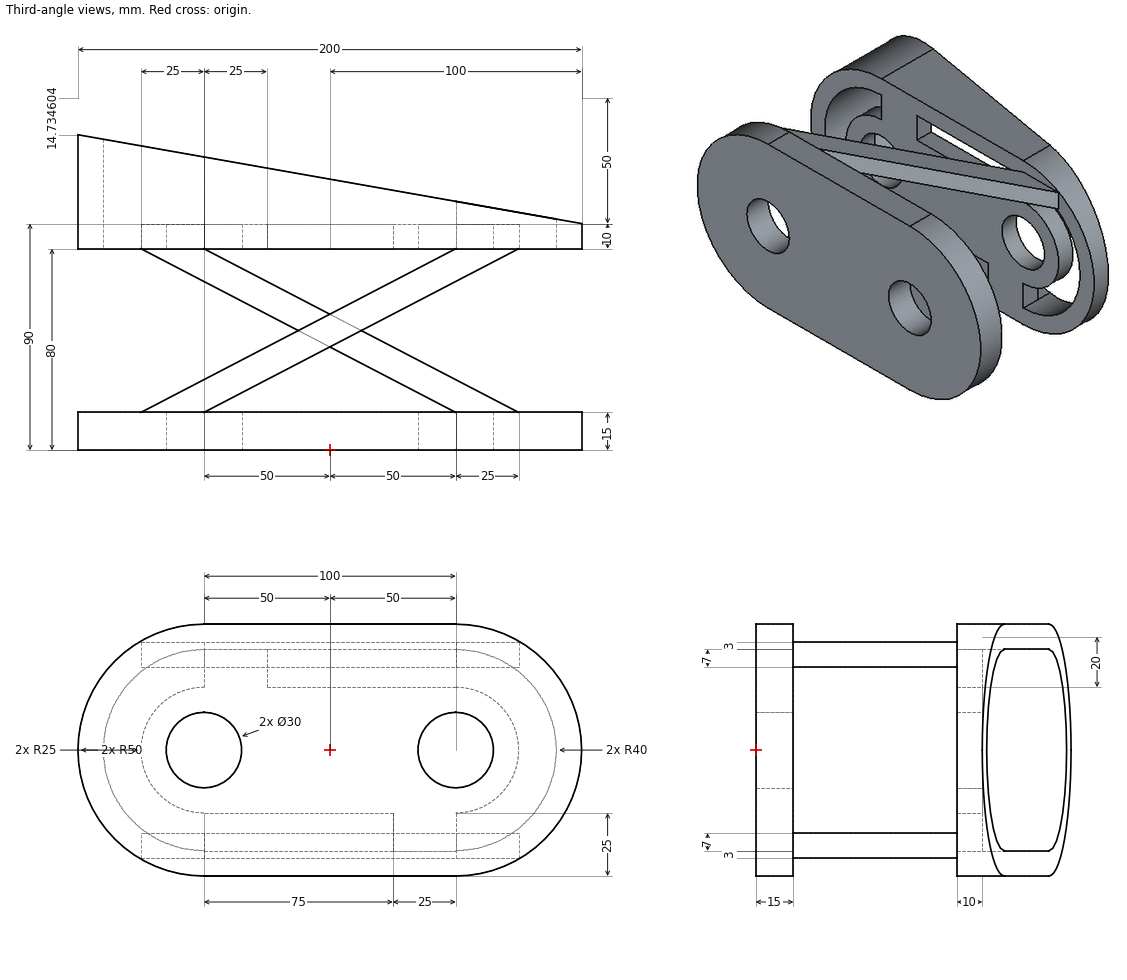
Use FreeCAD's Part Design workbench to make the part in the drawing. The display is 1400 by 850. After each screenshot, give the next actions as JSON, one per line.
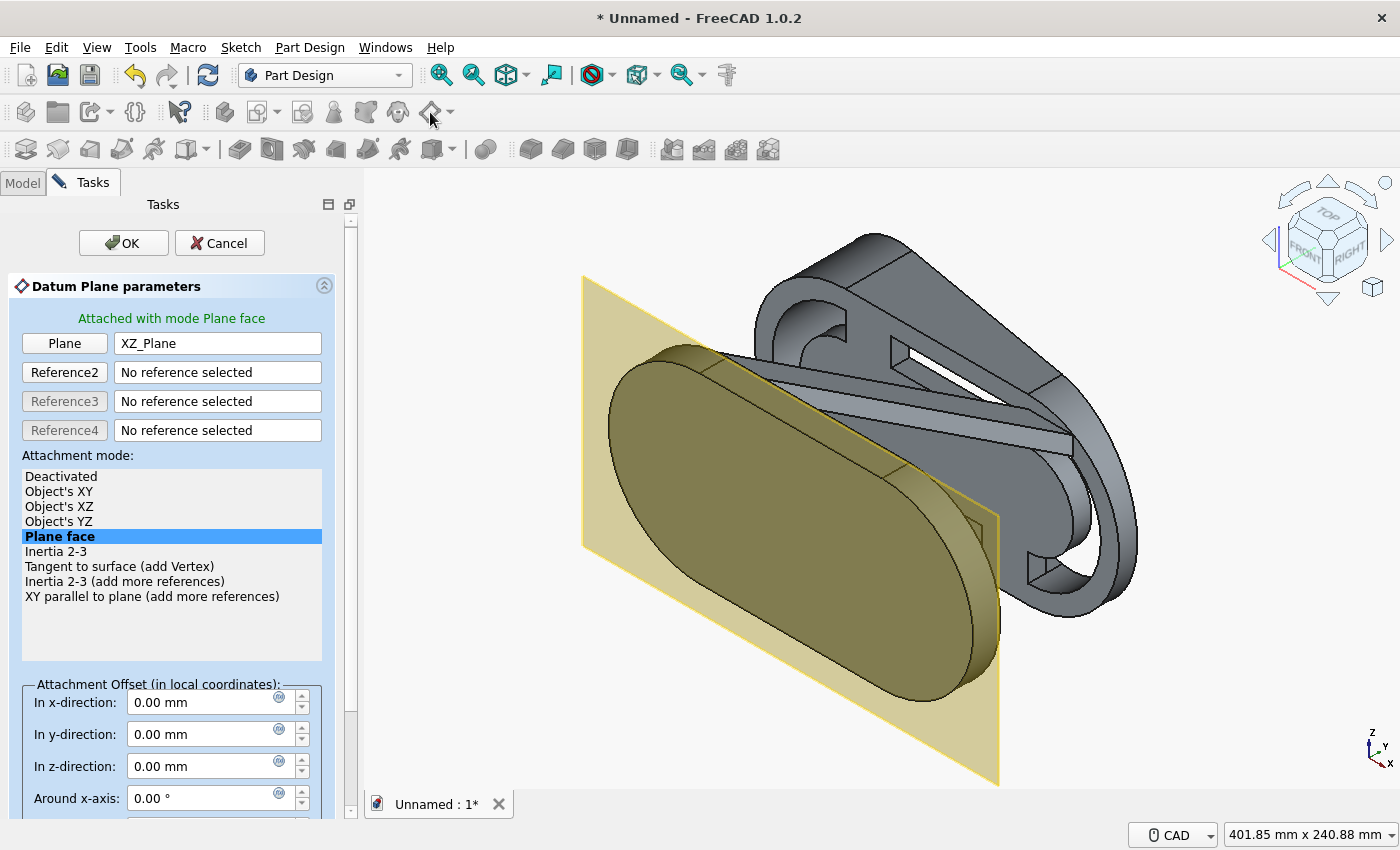
{"action": "triple_click", "coordinate": [210, 766]}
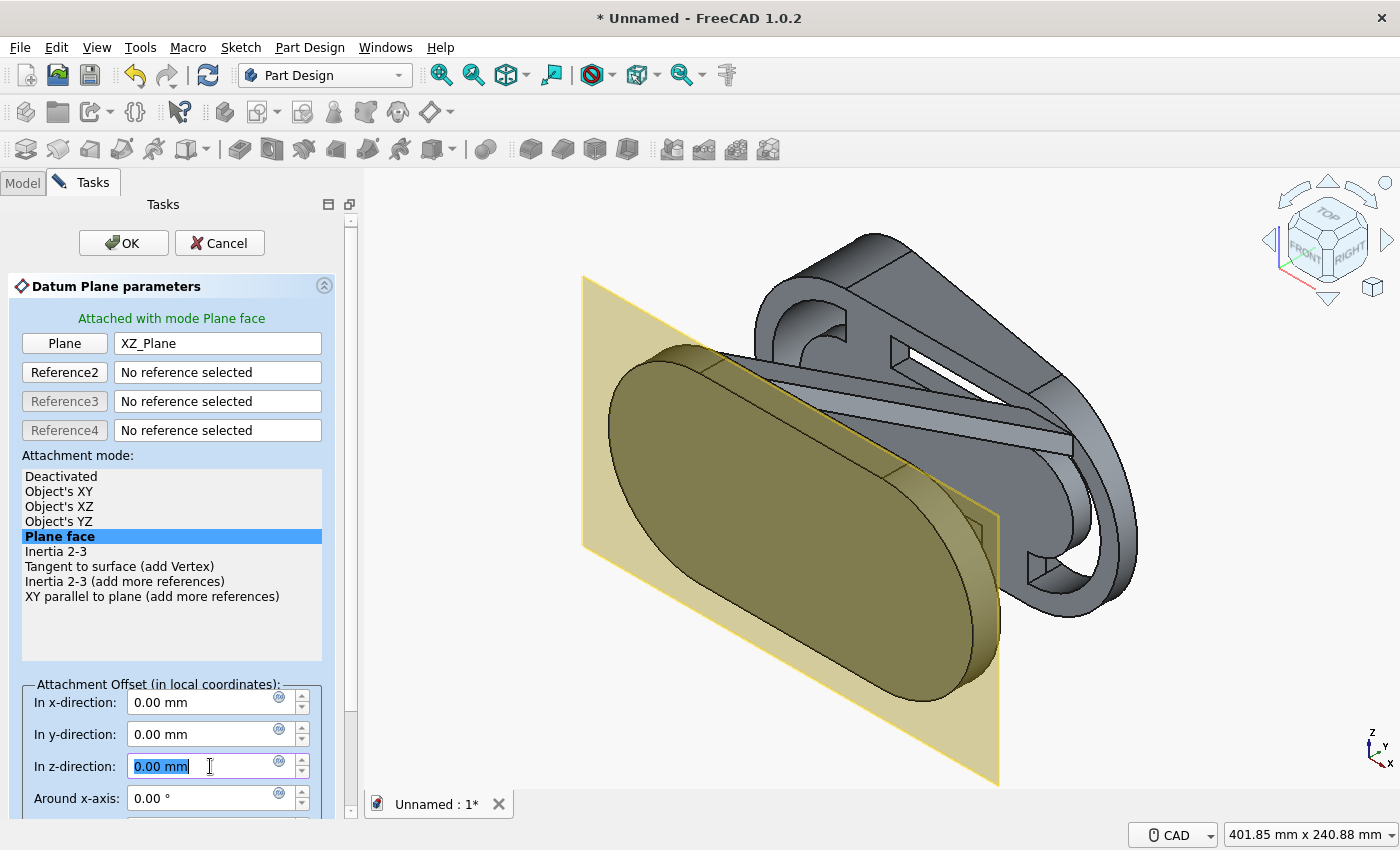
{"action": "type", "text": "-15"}
{"action": "key", "text": "Tab"}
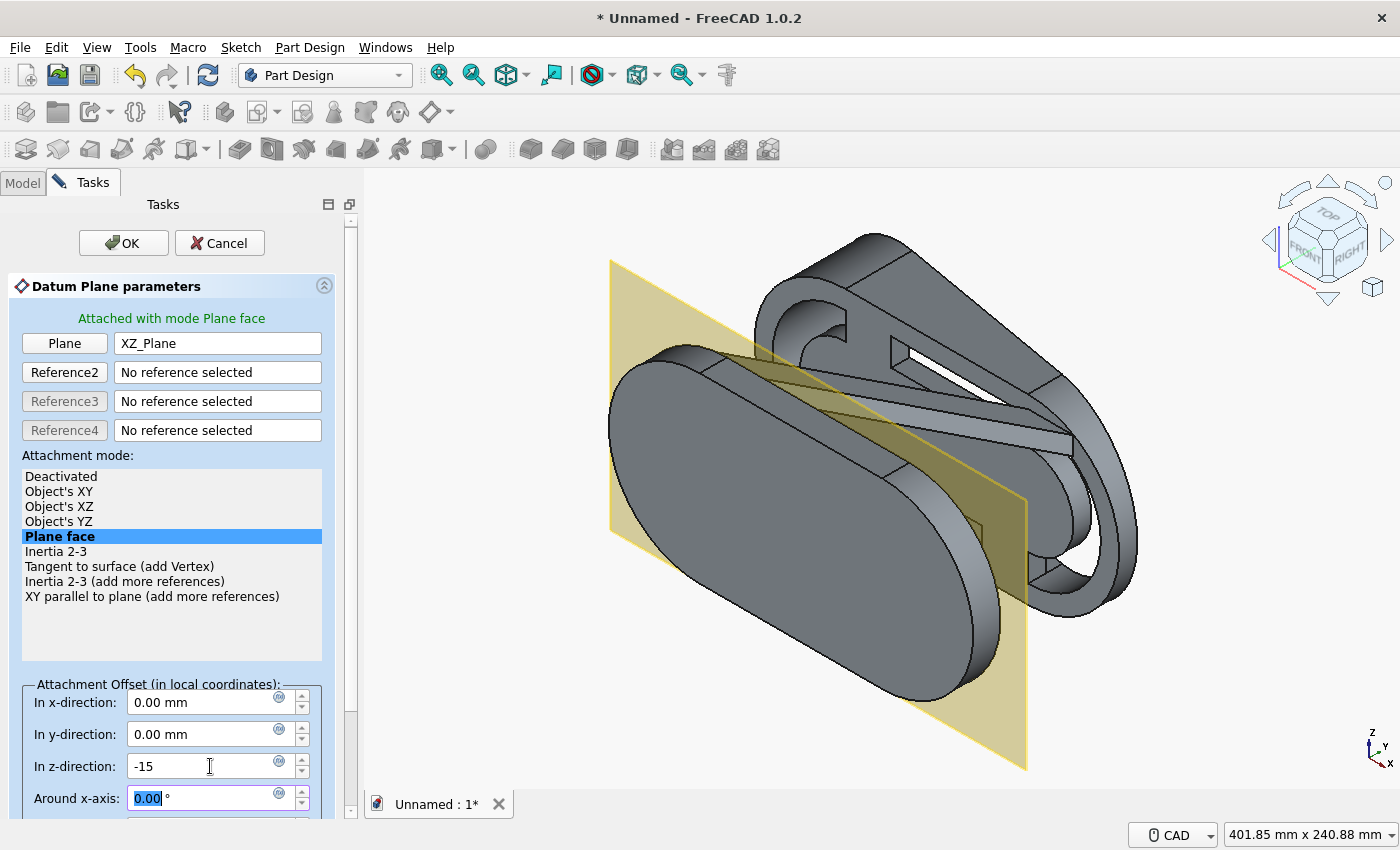
{"action": "left_click", "coordinate": [124, 243]}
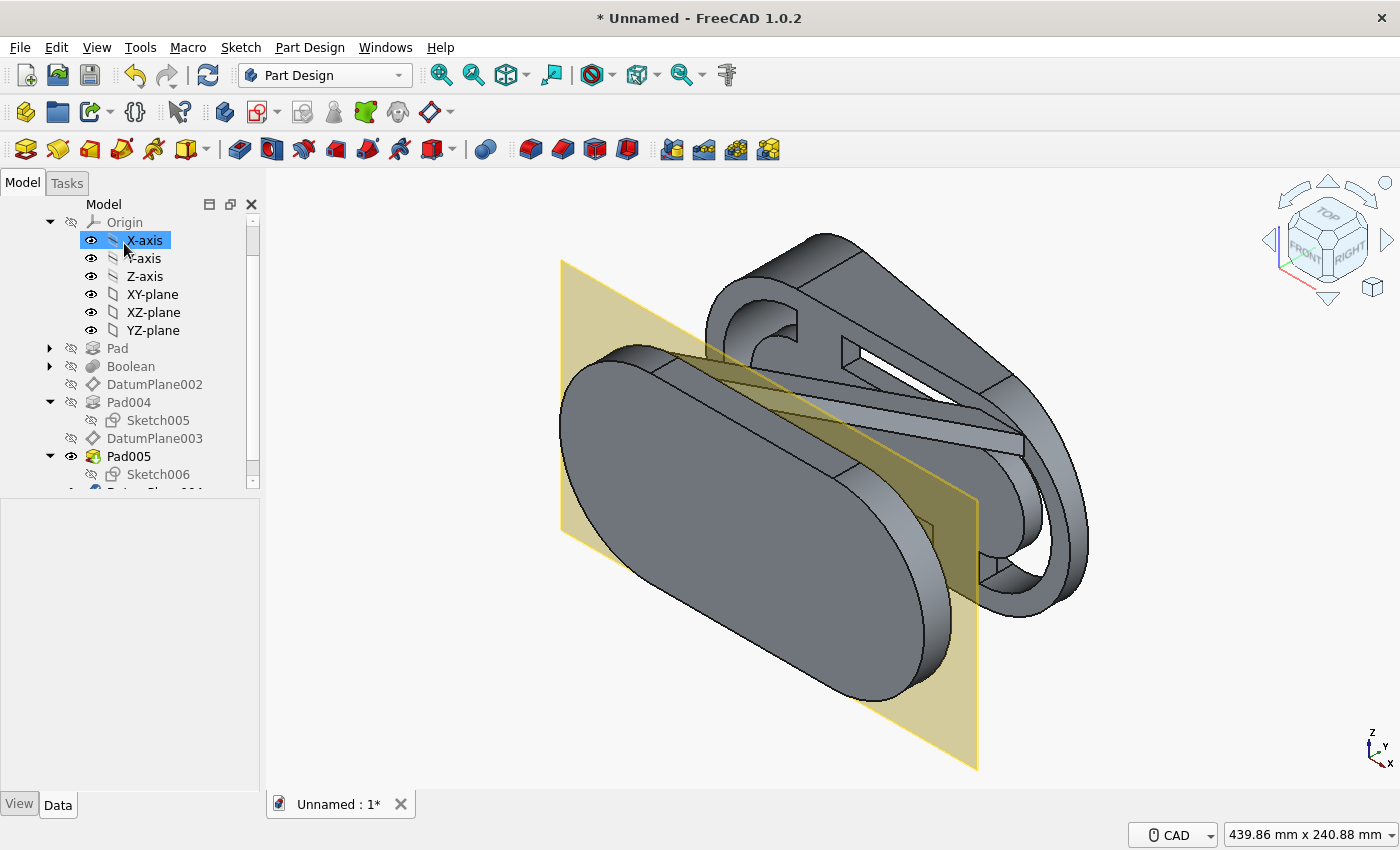
{"action": "scroll", "coordinate": [140, 344], "scroll_direction": "down", "scroll_amount": 3}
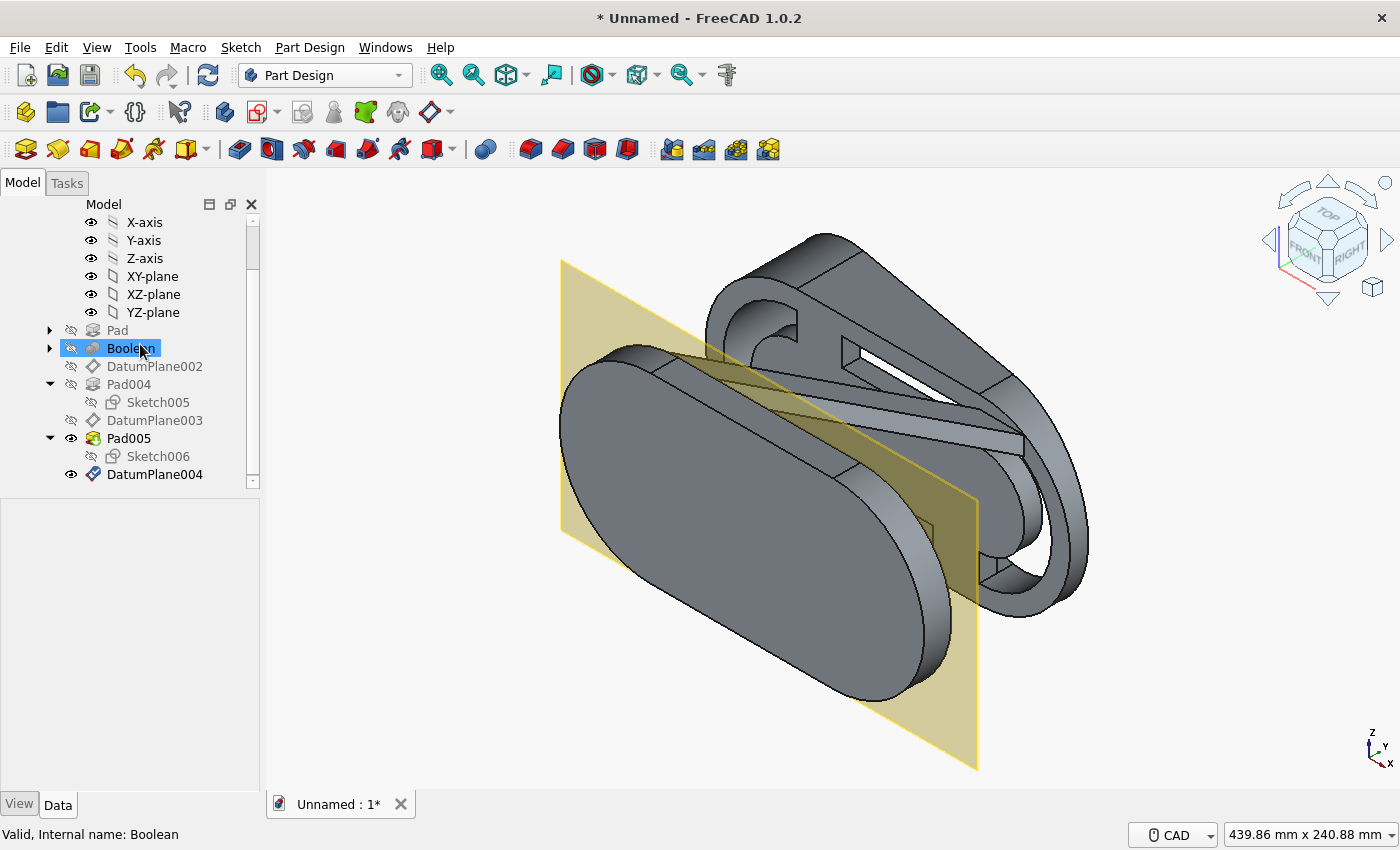
{"action": "left_click", "coordinate": [116, 474]}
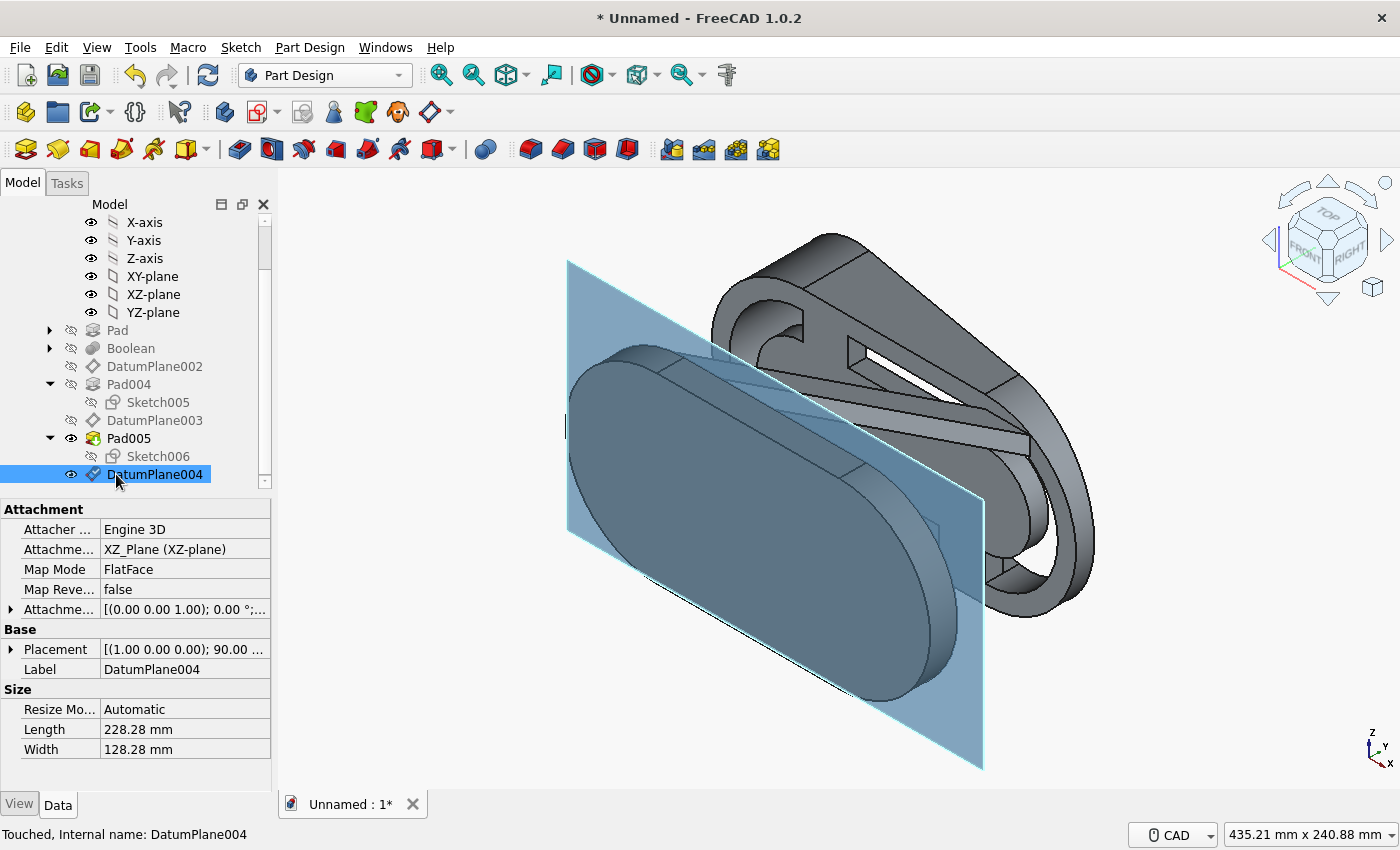
{"action": "left_click", "coordinate": [258, 112]}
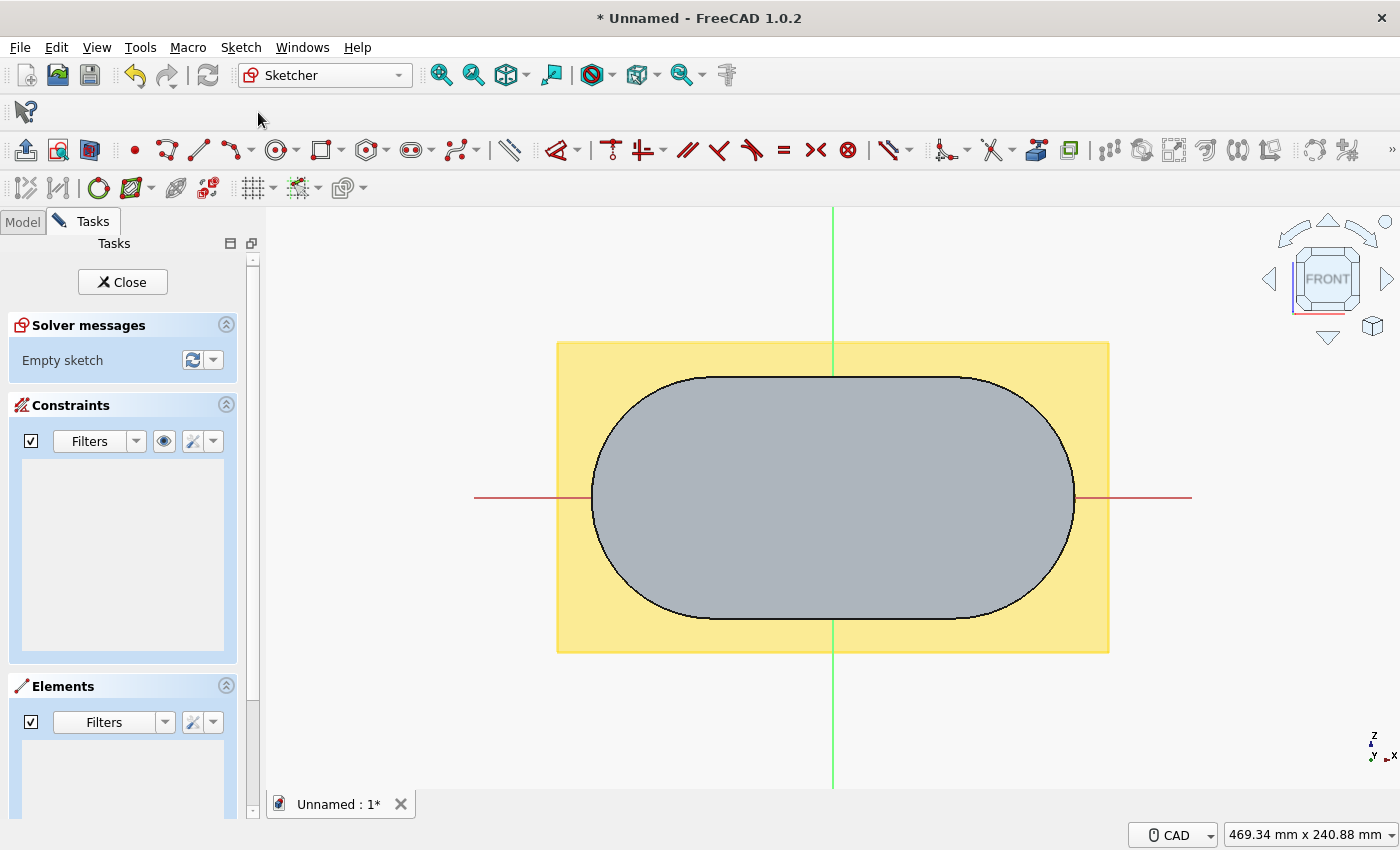
{"action": "left_click", "coordinate": [90, 150]}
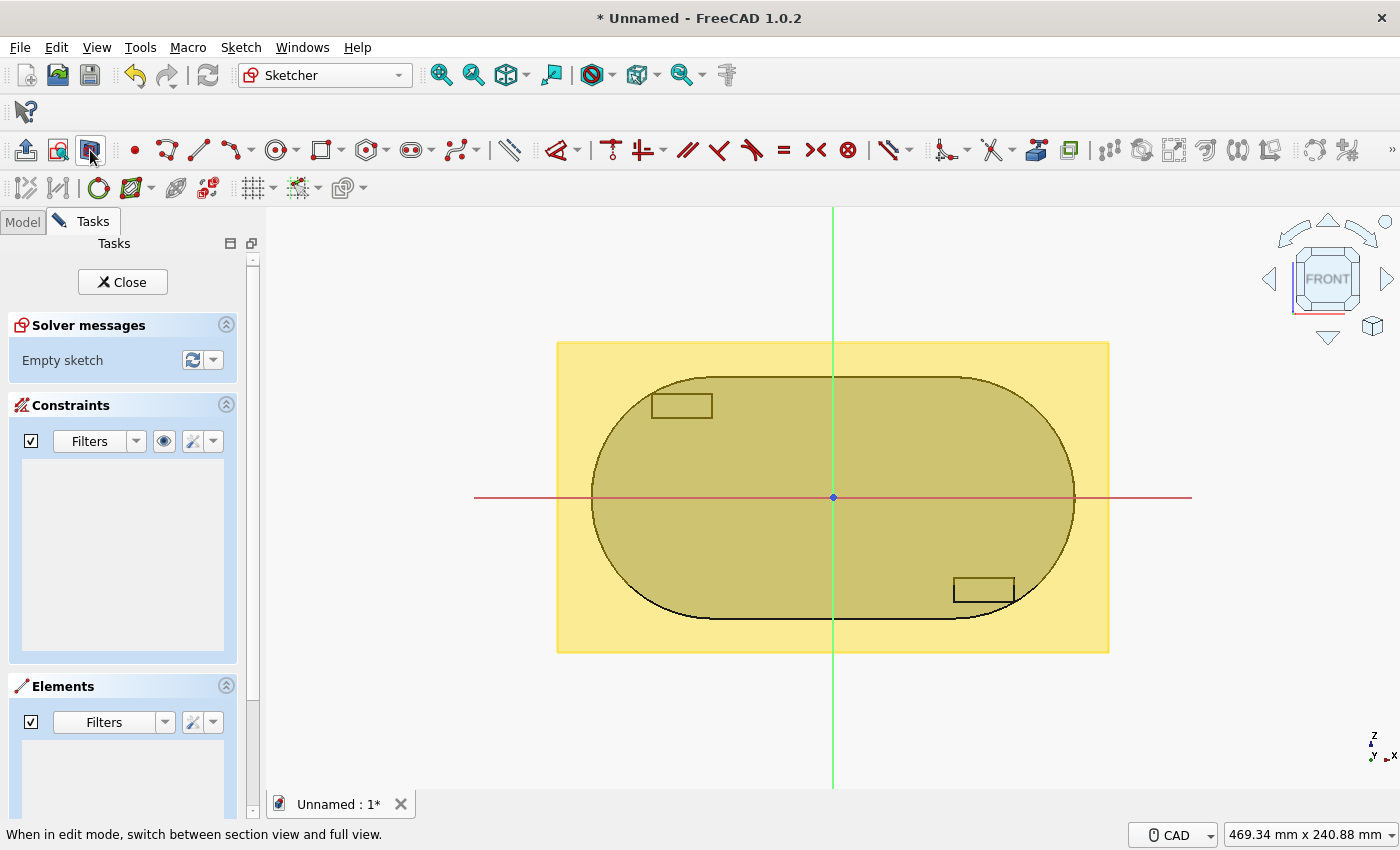
{"action": "scroll", "coordinate": [889, 498], "scroll_direction": "up", "scroll_amount": 4}